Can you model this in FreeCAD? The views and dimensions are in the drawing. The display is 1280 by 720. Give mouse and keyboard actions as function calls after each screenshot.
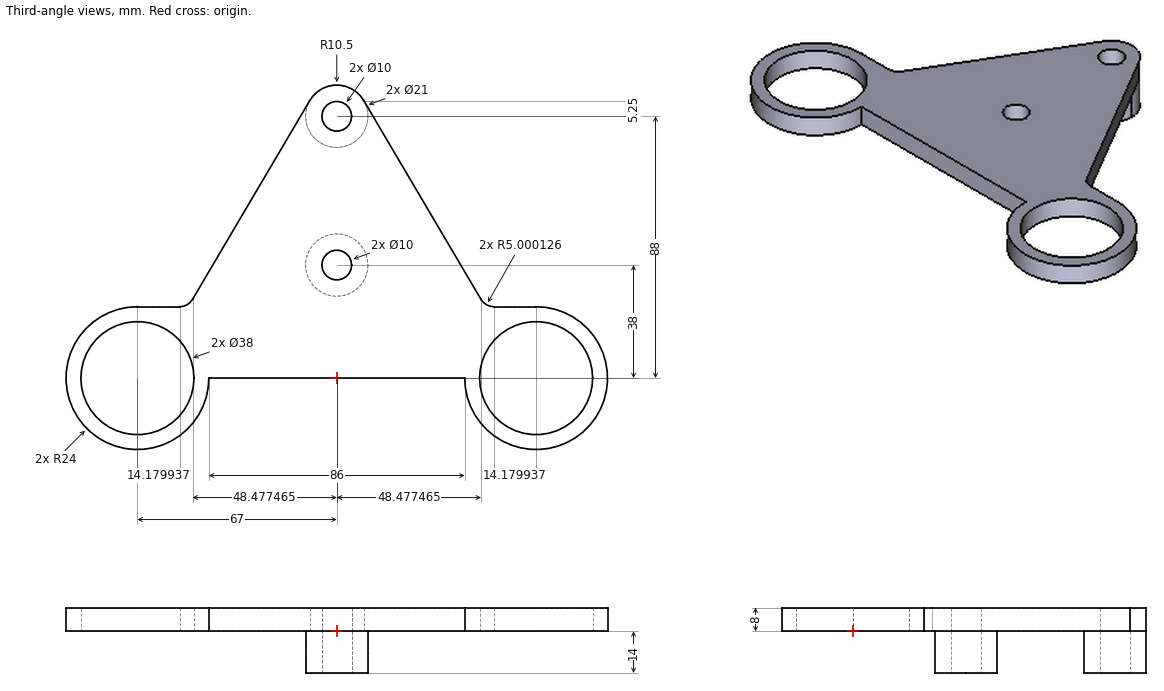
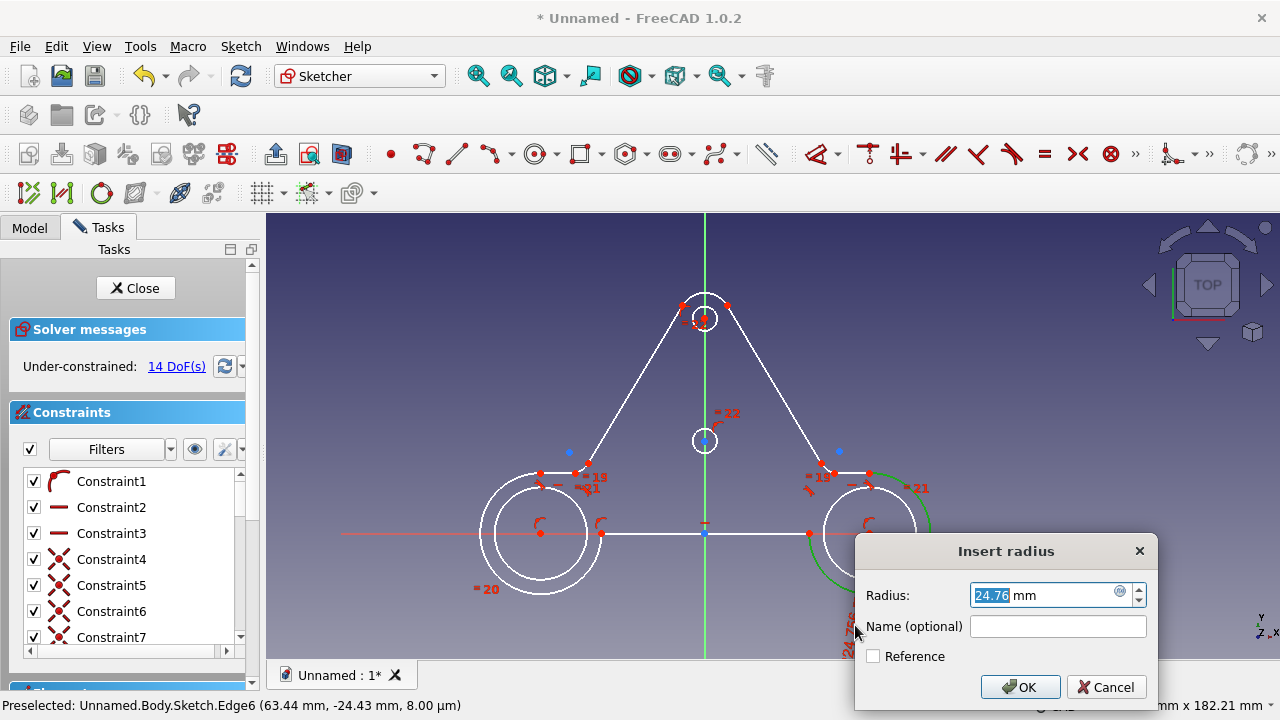
text(24)
key(Return)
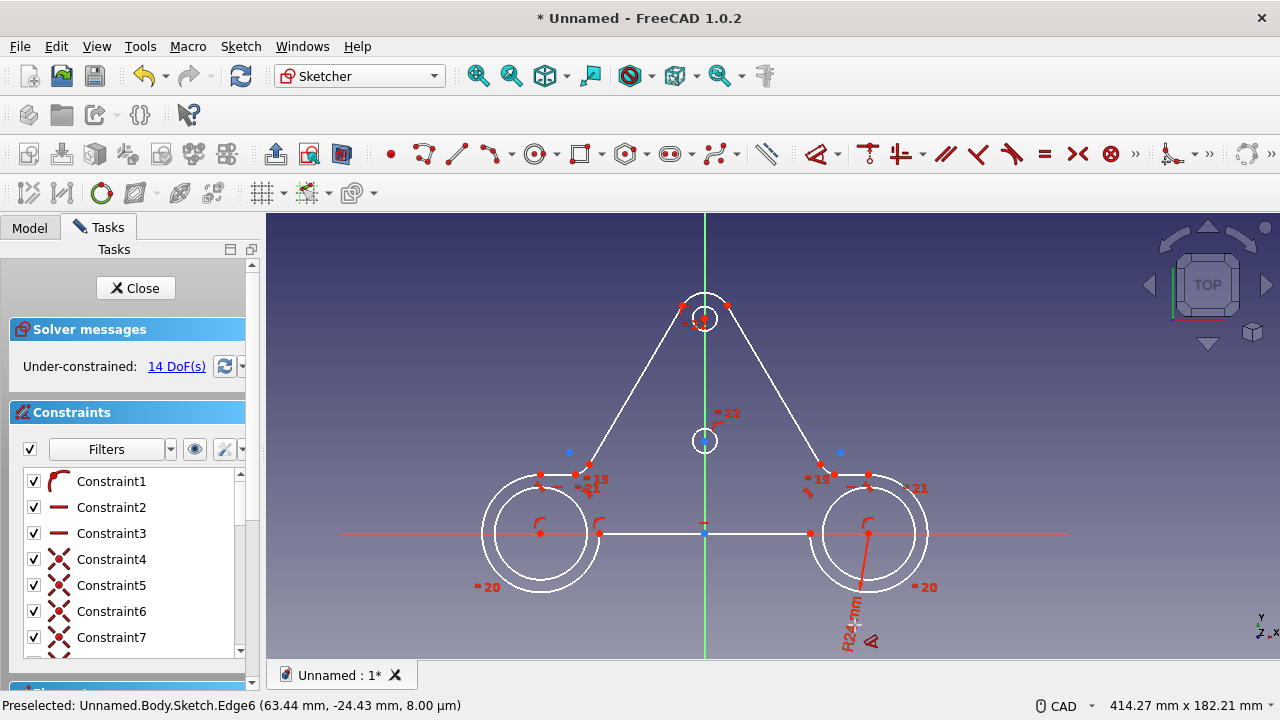
scroll(826, 471, up, 6)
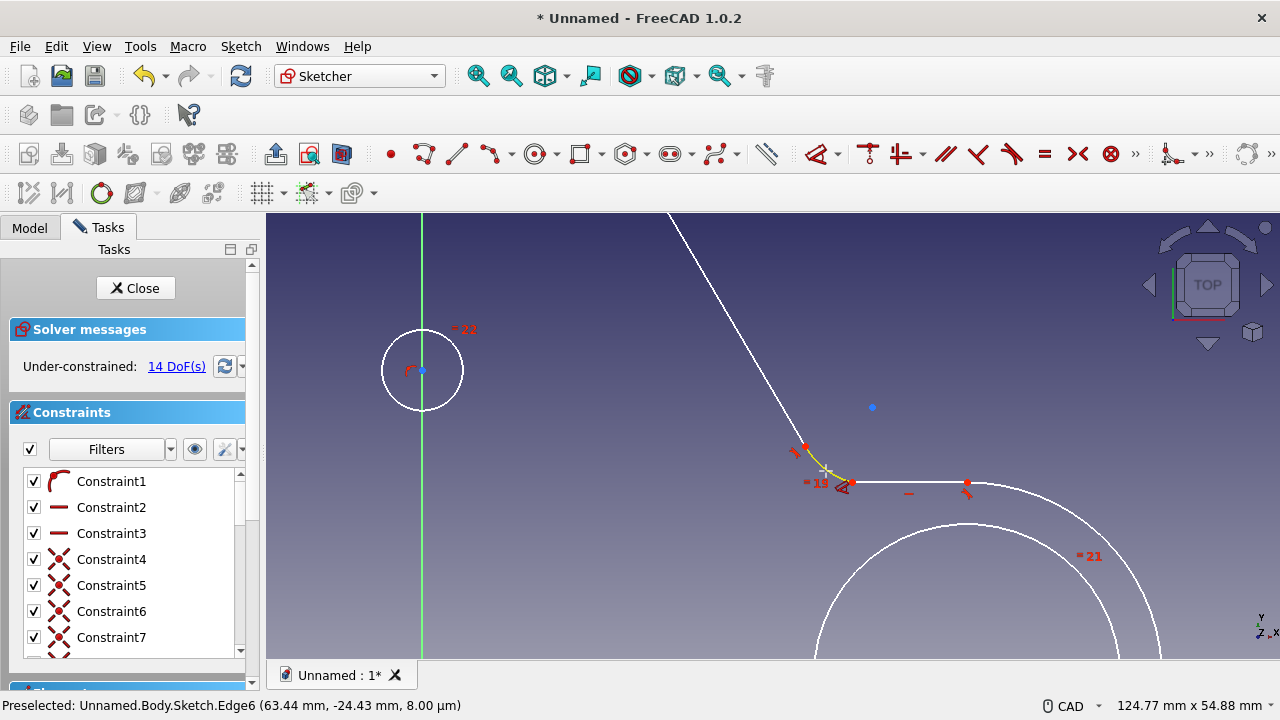
click(825, 469)
click(805, 494)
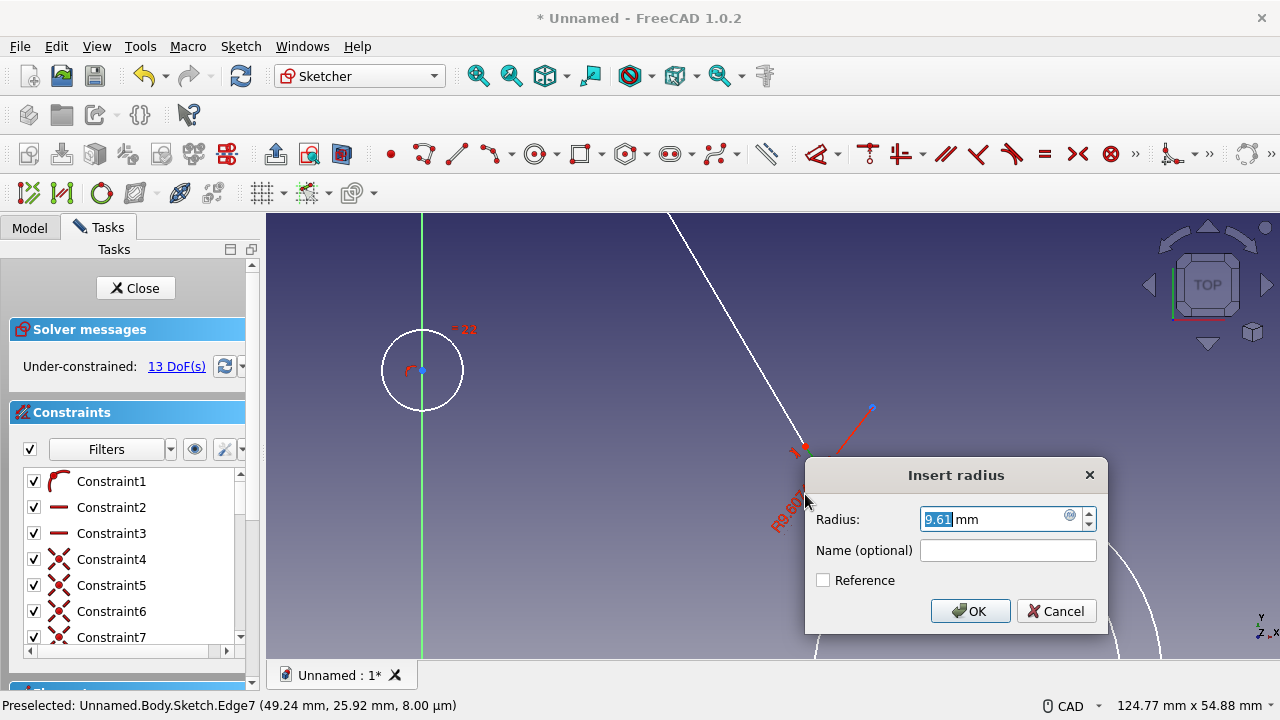
text(5.000126)
key(Return)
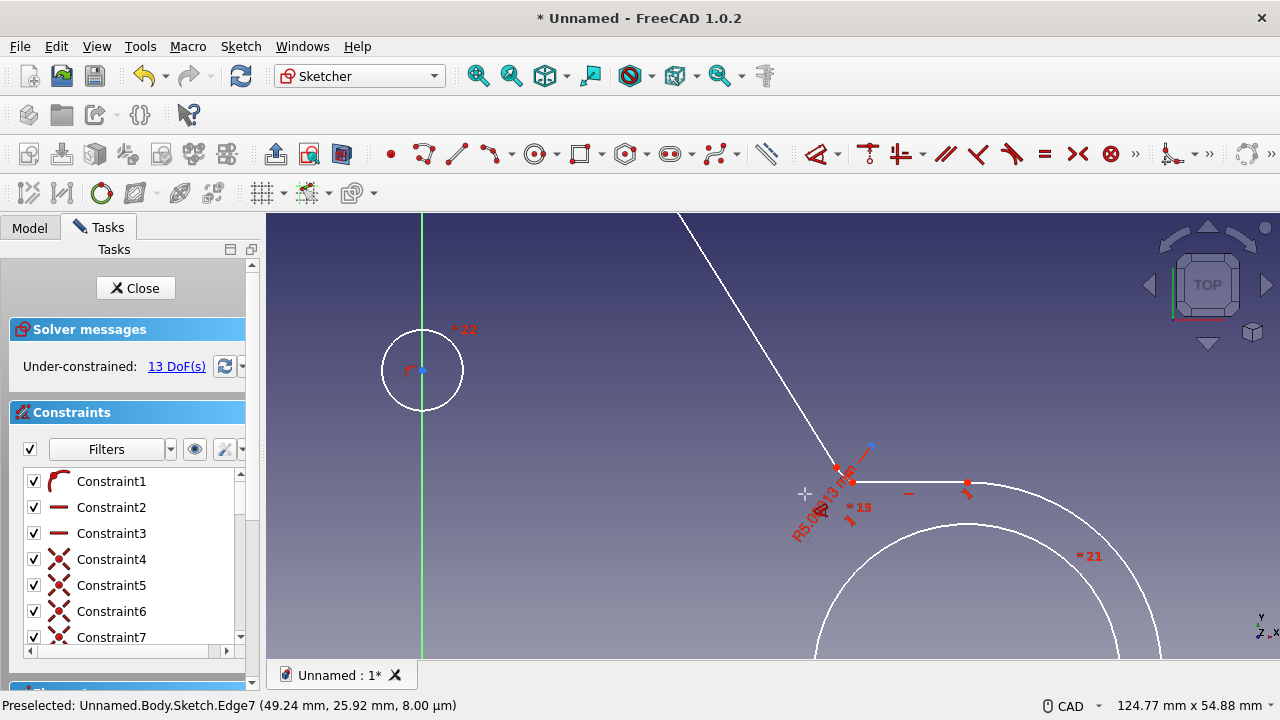
scroll(826, 471, down, 6)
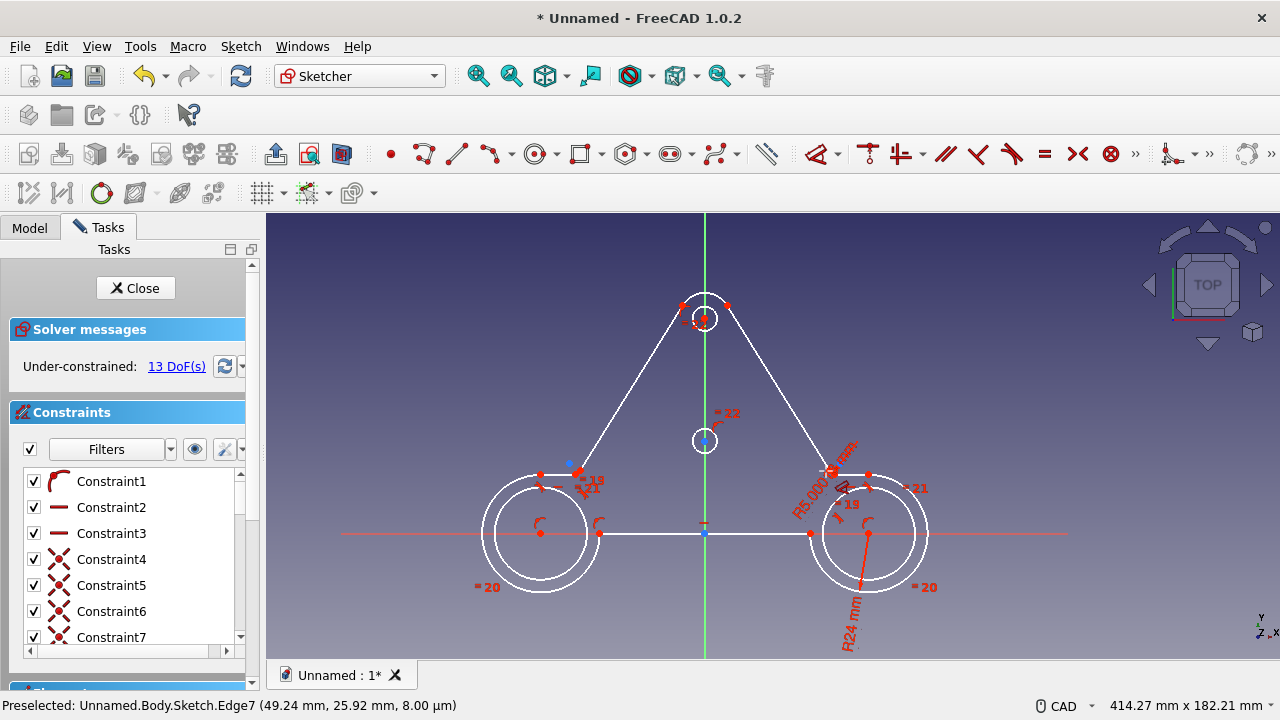
scroll(715, 295, up, 3)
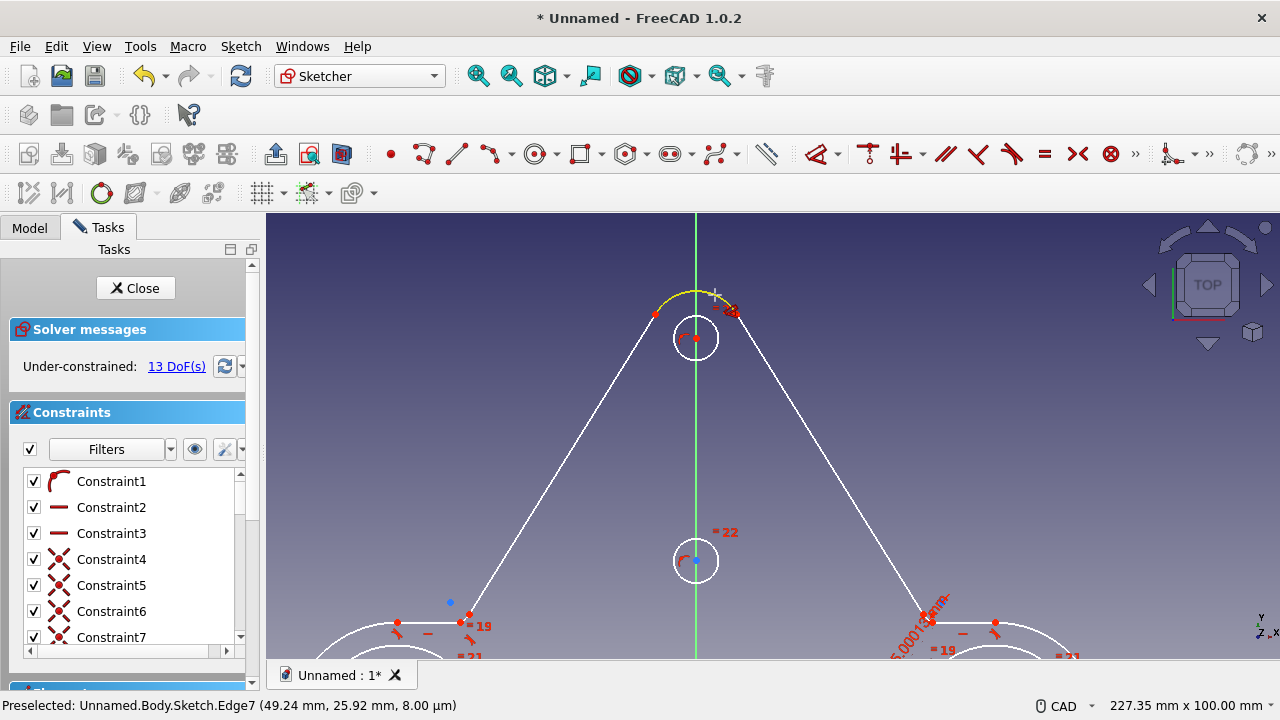
click(715, 295)
click(728, 266)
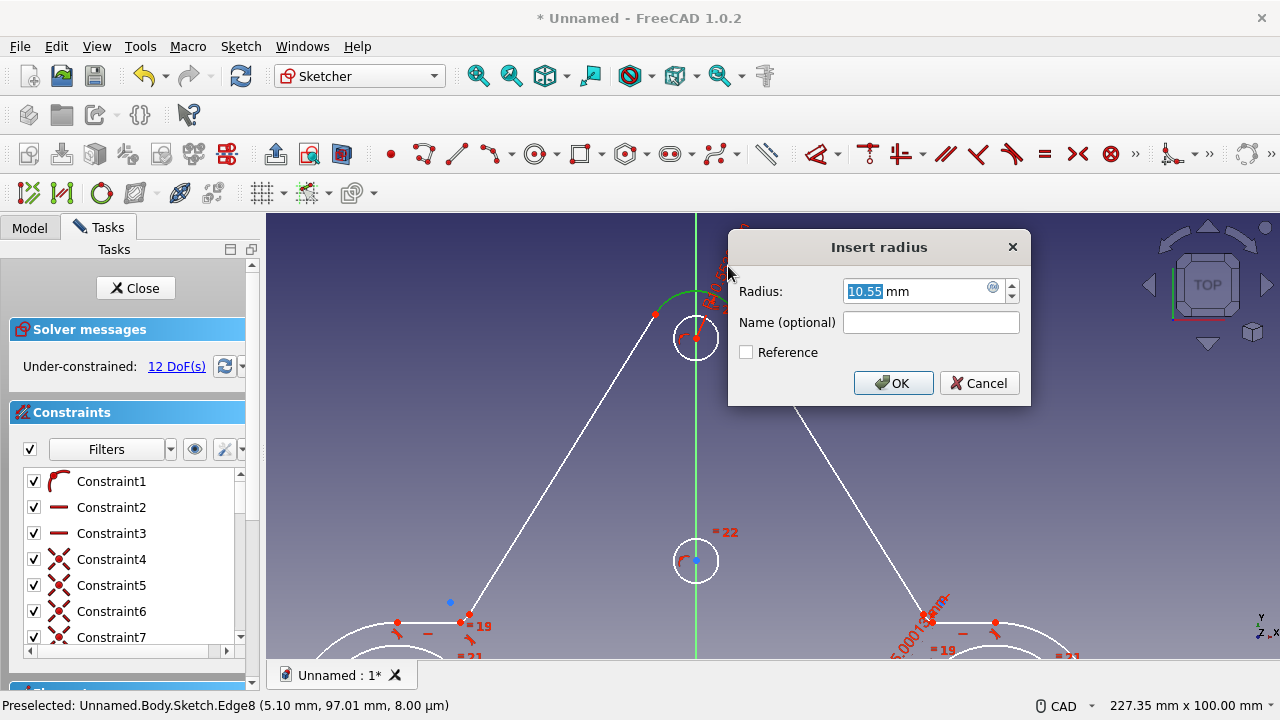
text(10.5)
key(Return)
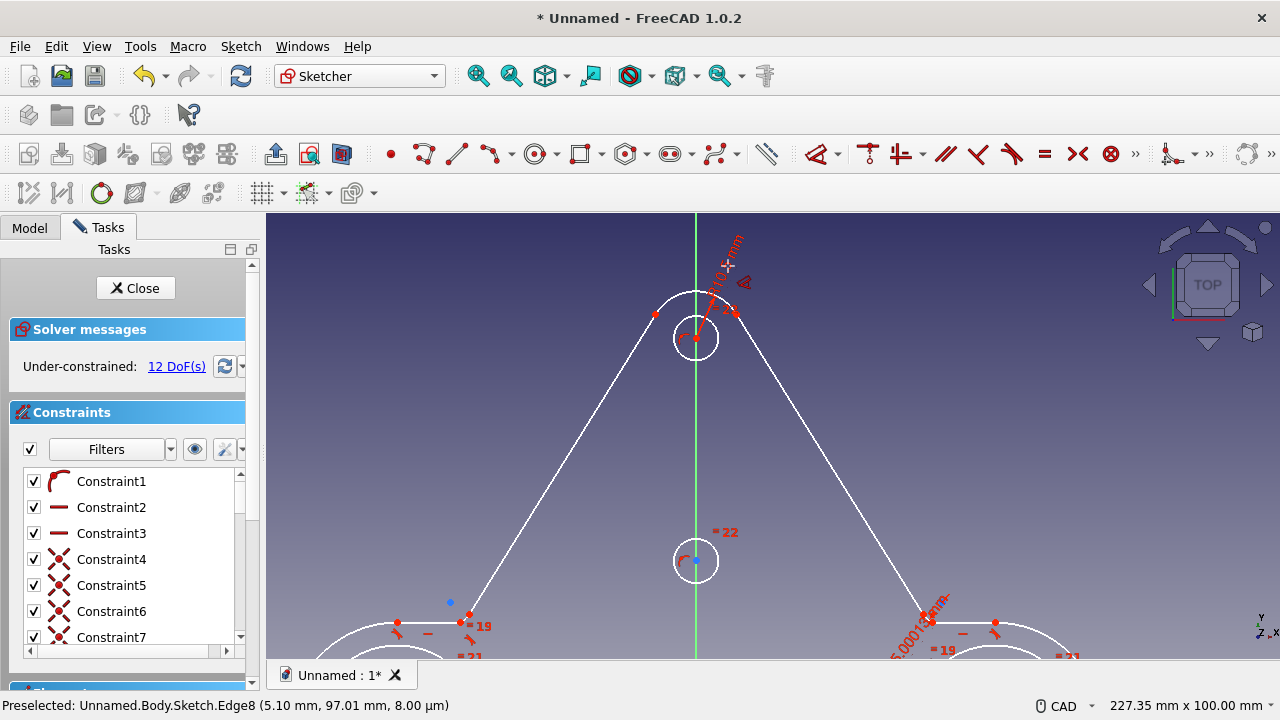
scroll(715, 295, down, 3)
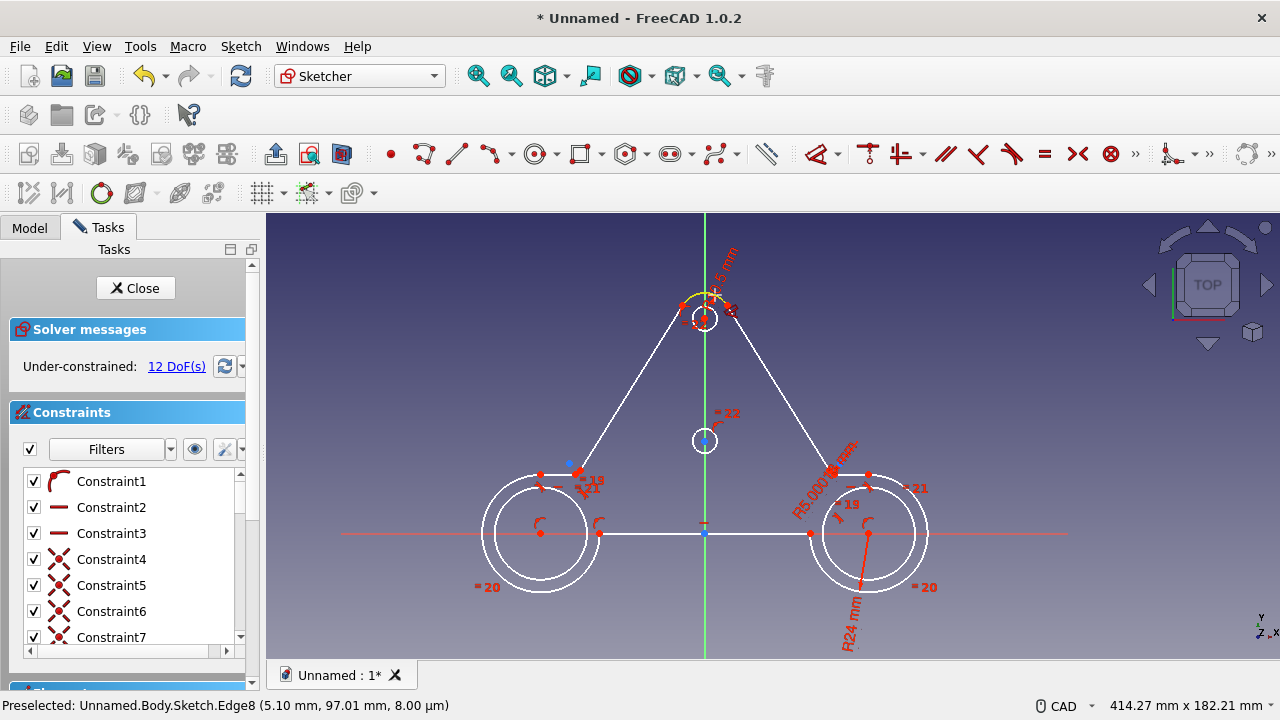
click(573, 501)
click(595, 478)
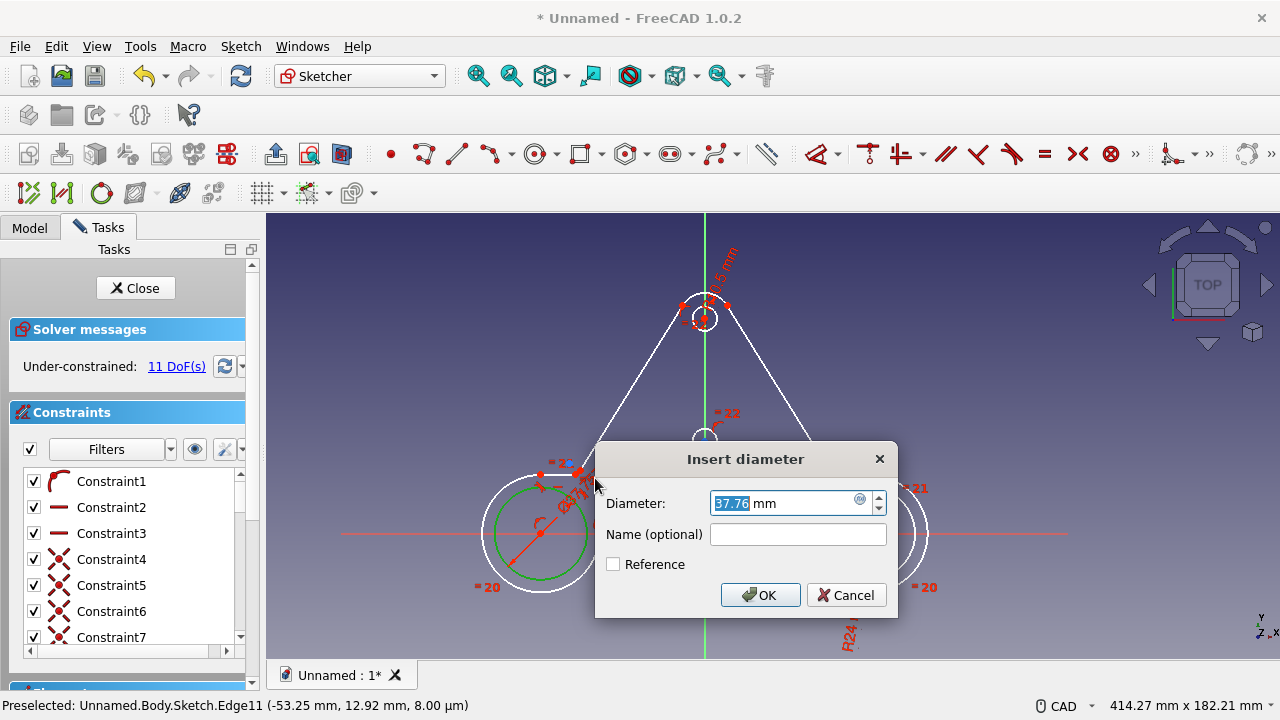
text(38)
key(Return)